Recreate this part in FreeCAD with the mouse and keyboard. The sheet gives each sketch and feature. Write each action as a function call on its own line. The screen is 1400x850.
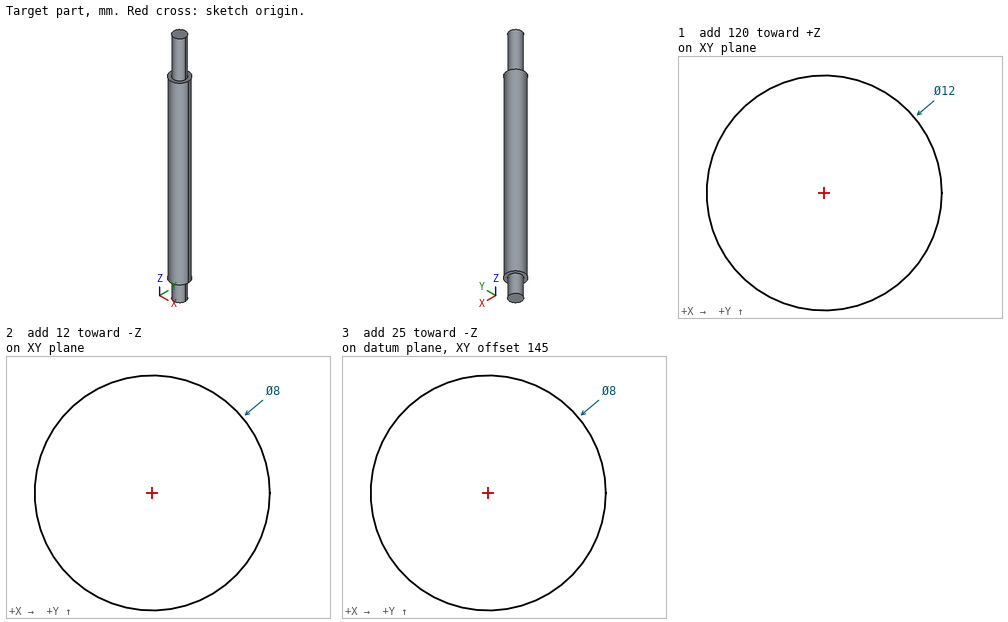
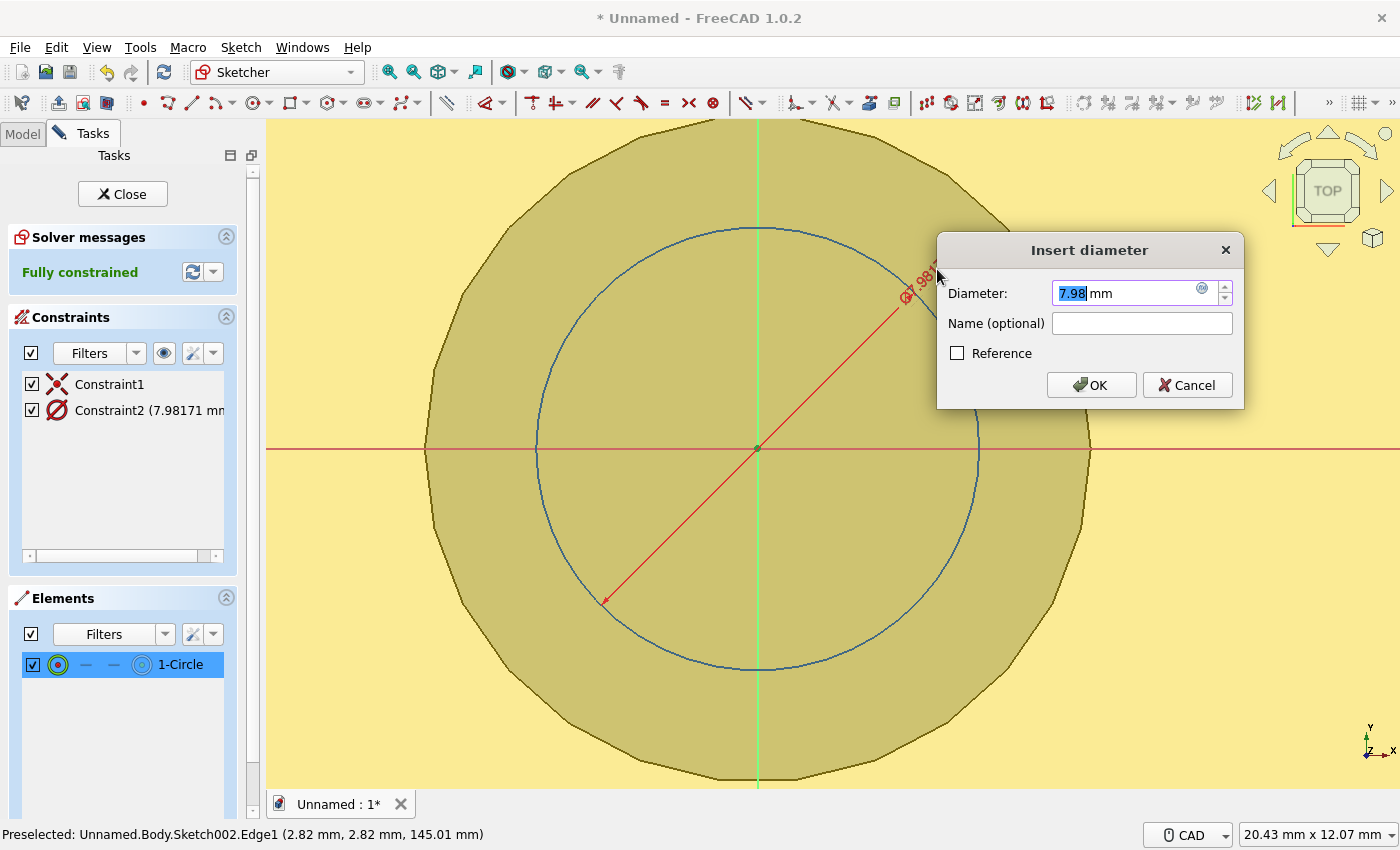
text(8)
key(Return)
key(Escape)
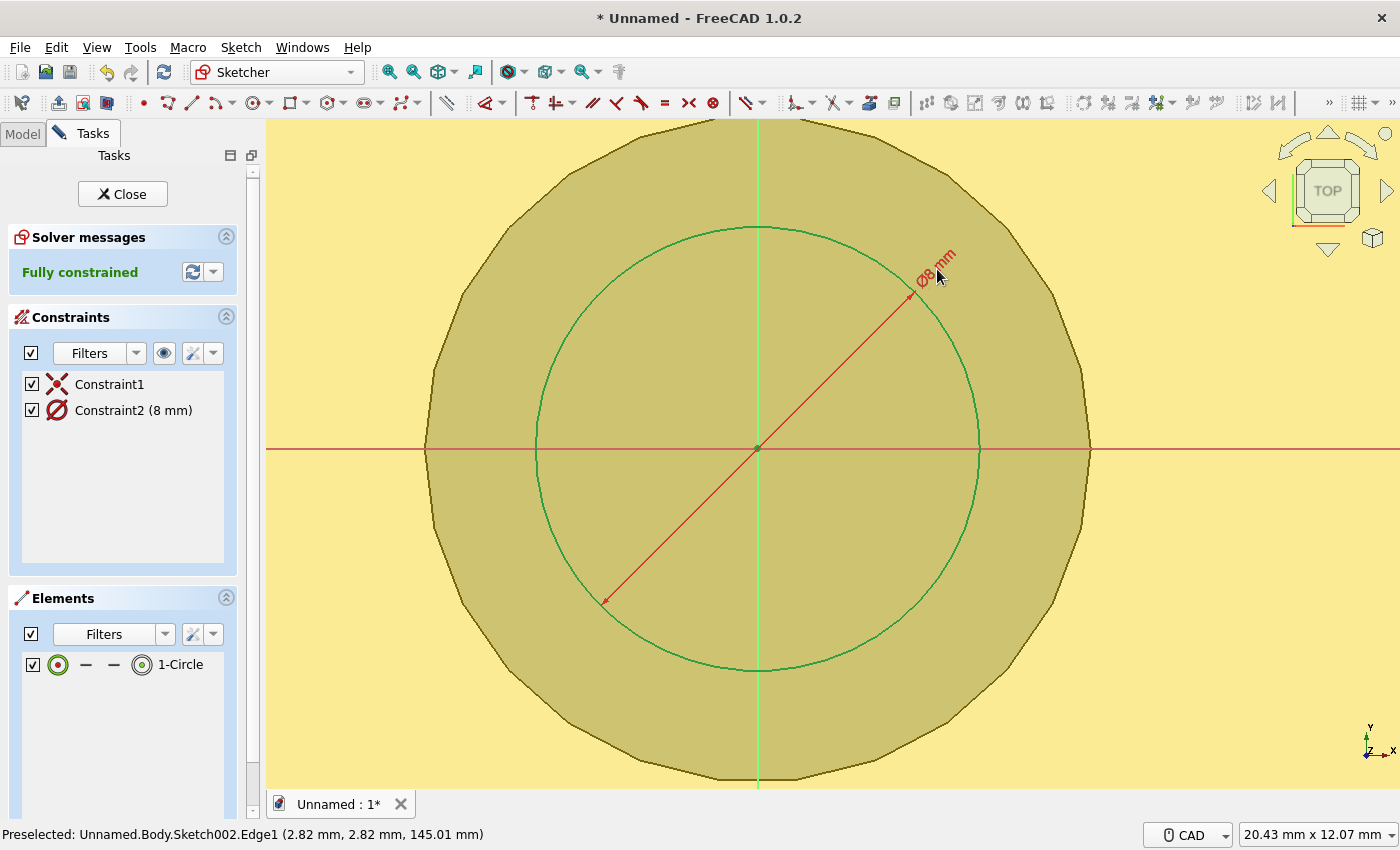
click(123, 194)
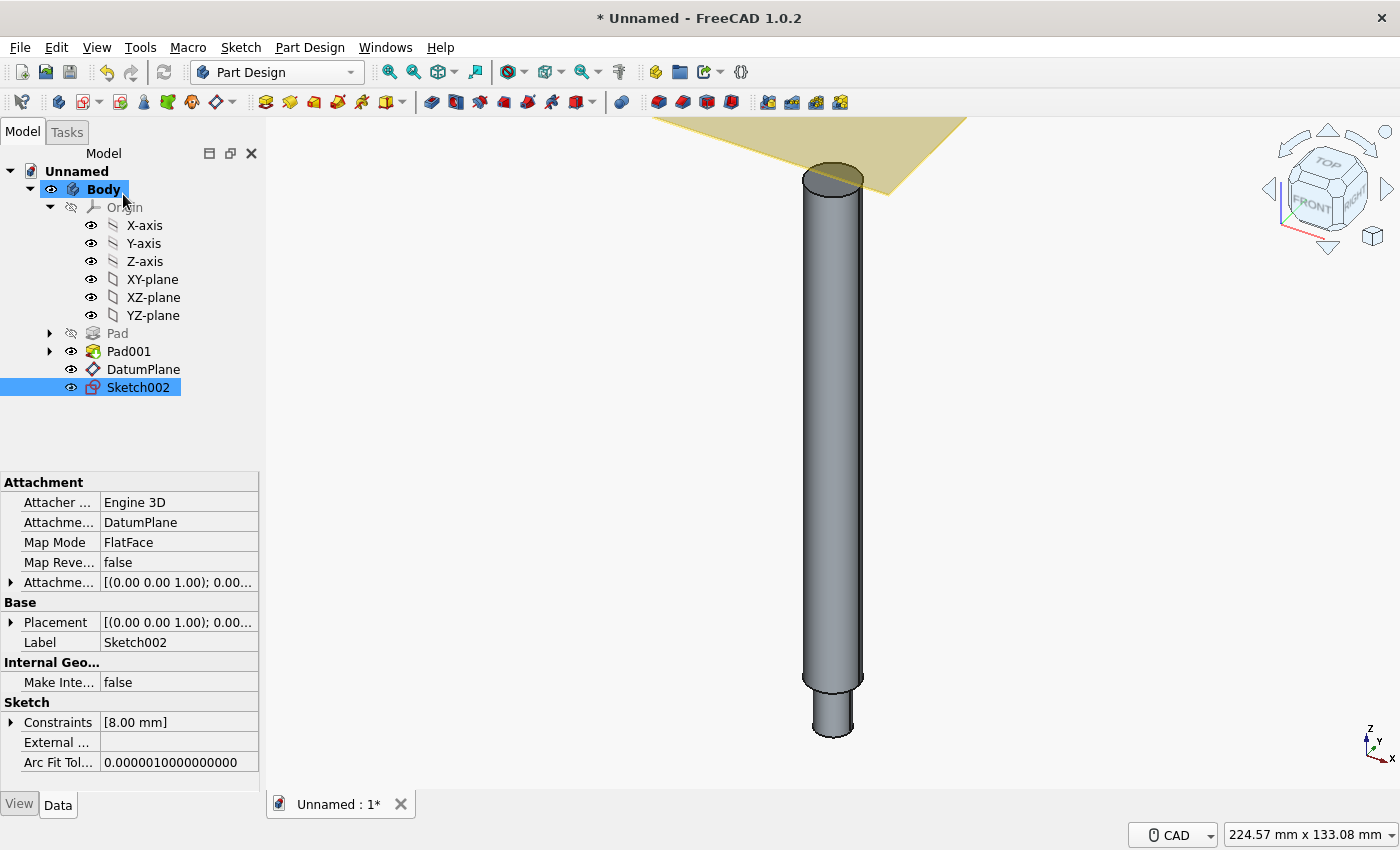
click(266, 102)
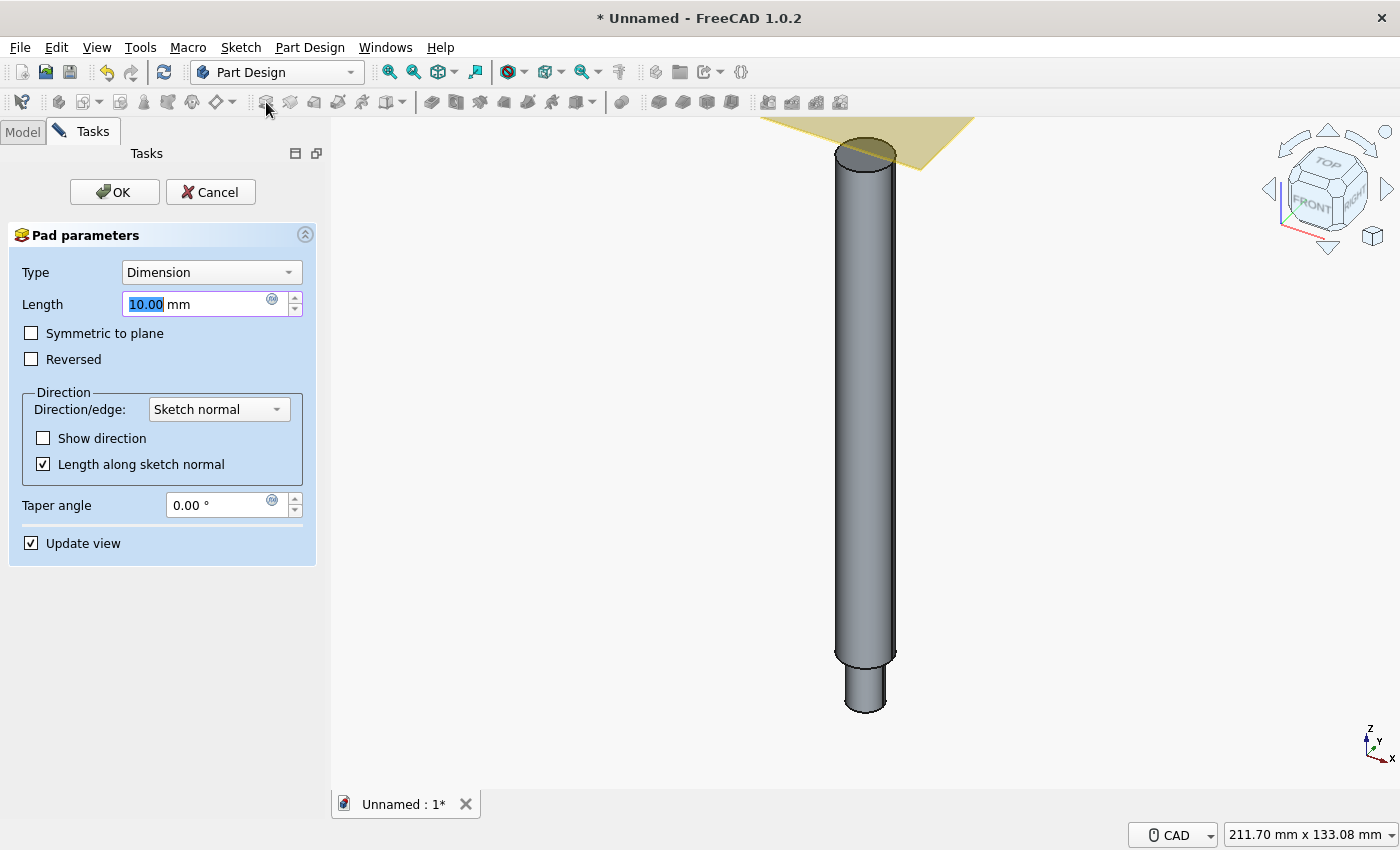
text(25)
key(Tab)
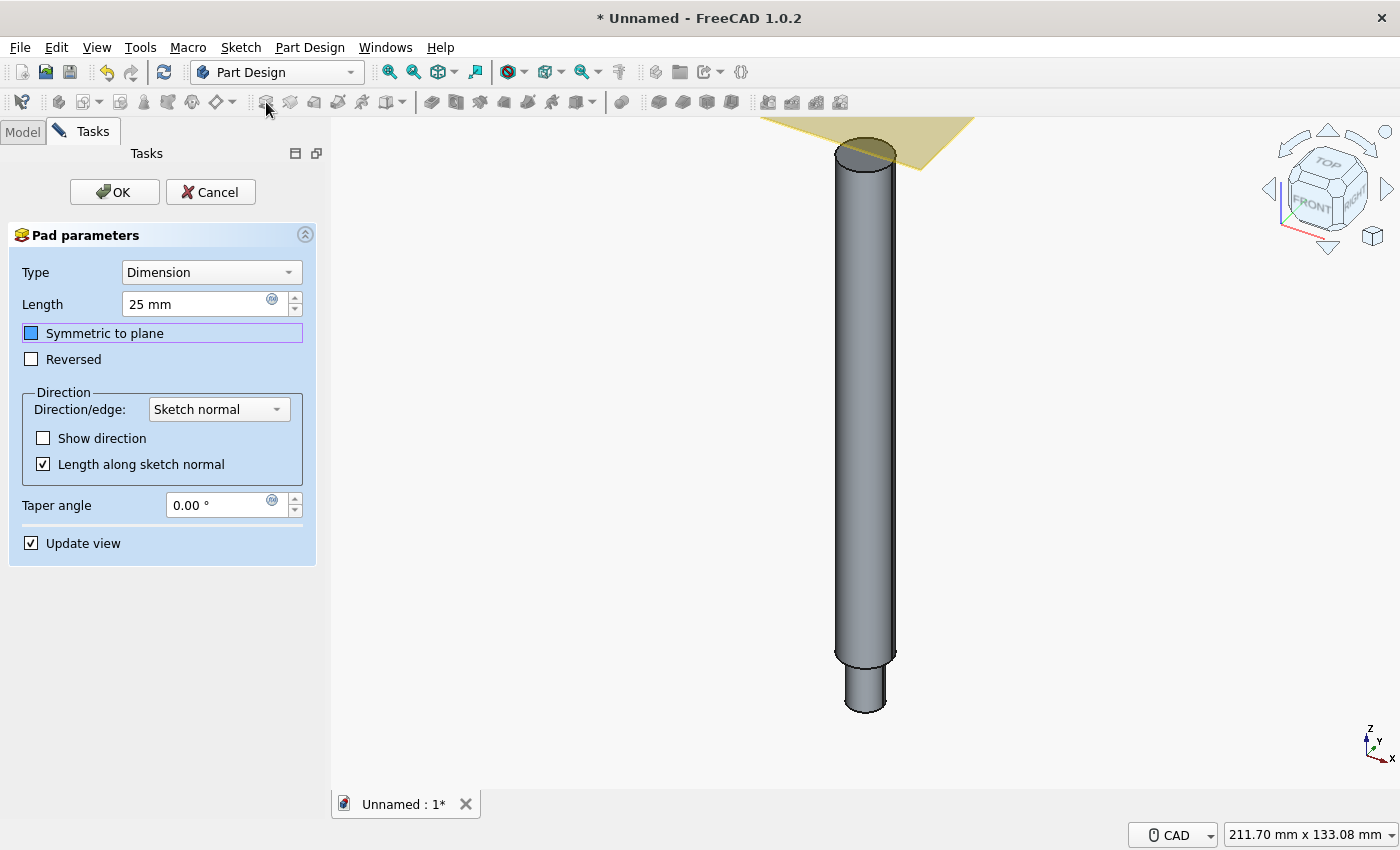
click(30, 359)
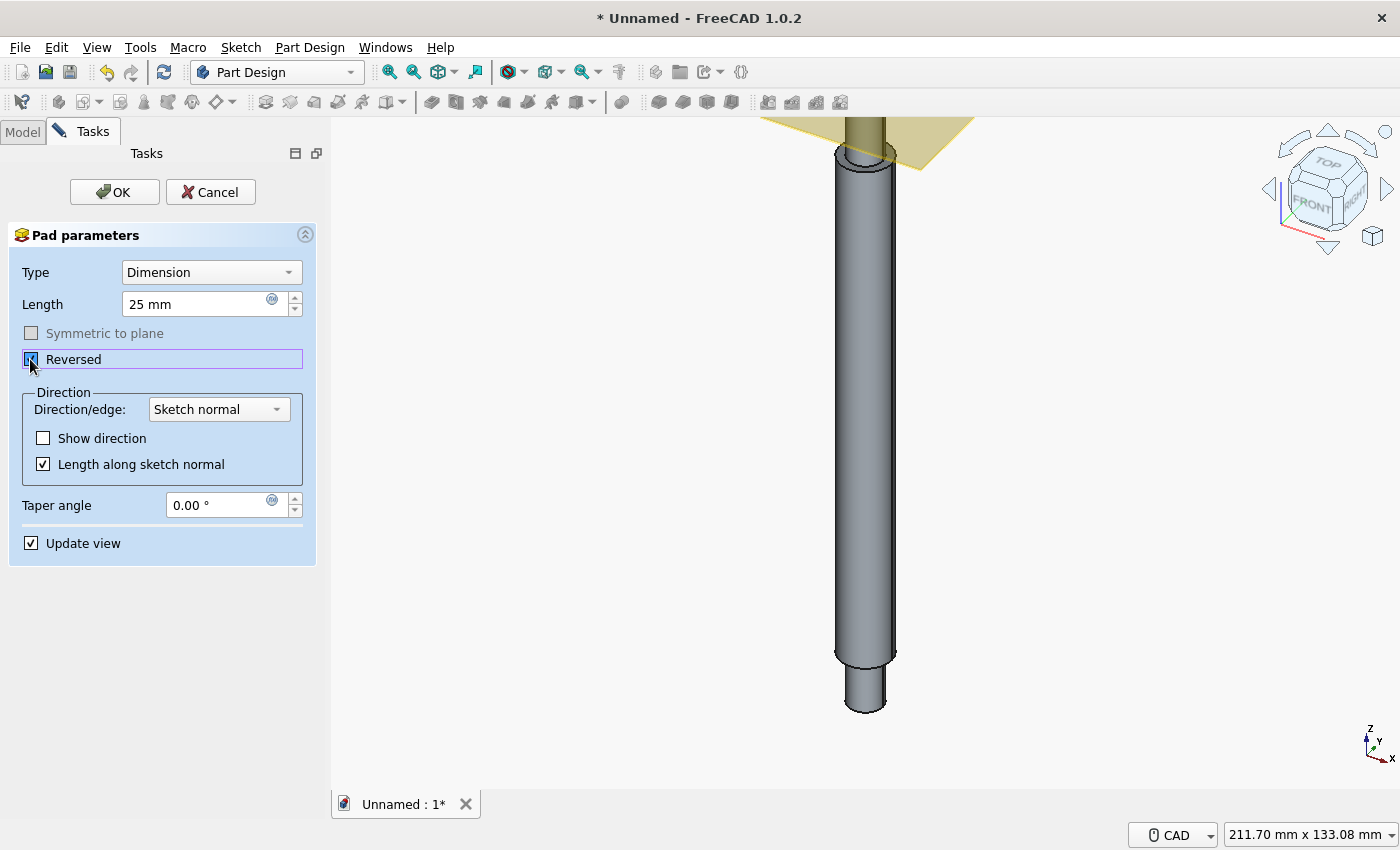
click(115, 192)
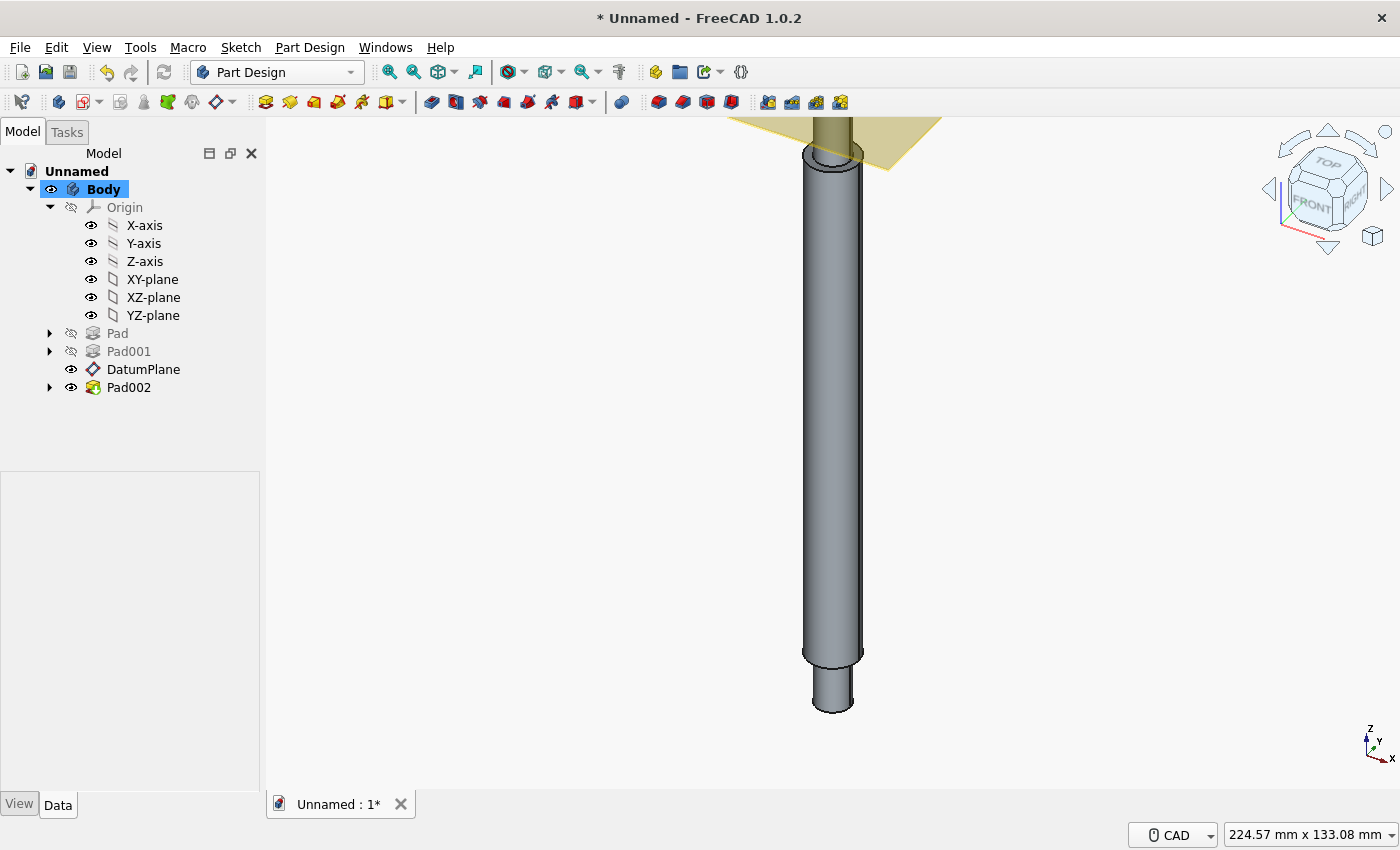
click(116, 369)
key(space)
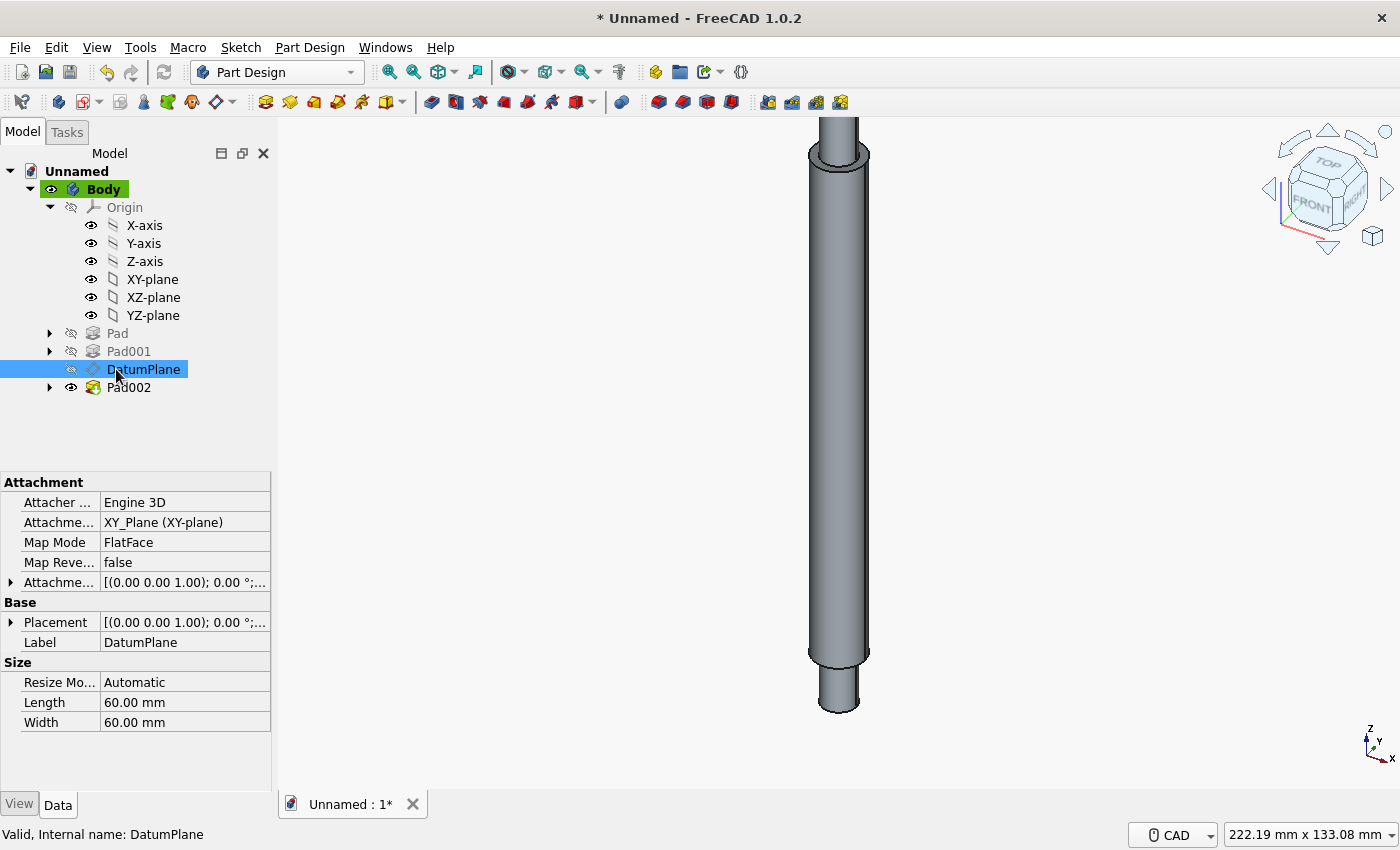
key(0)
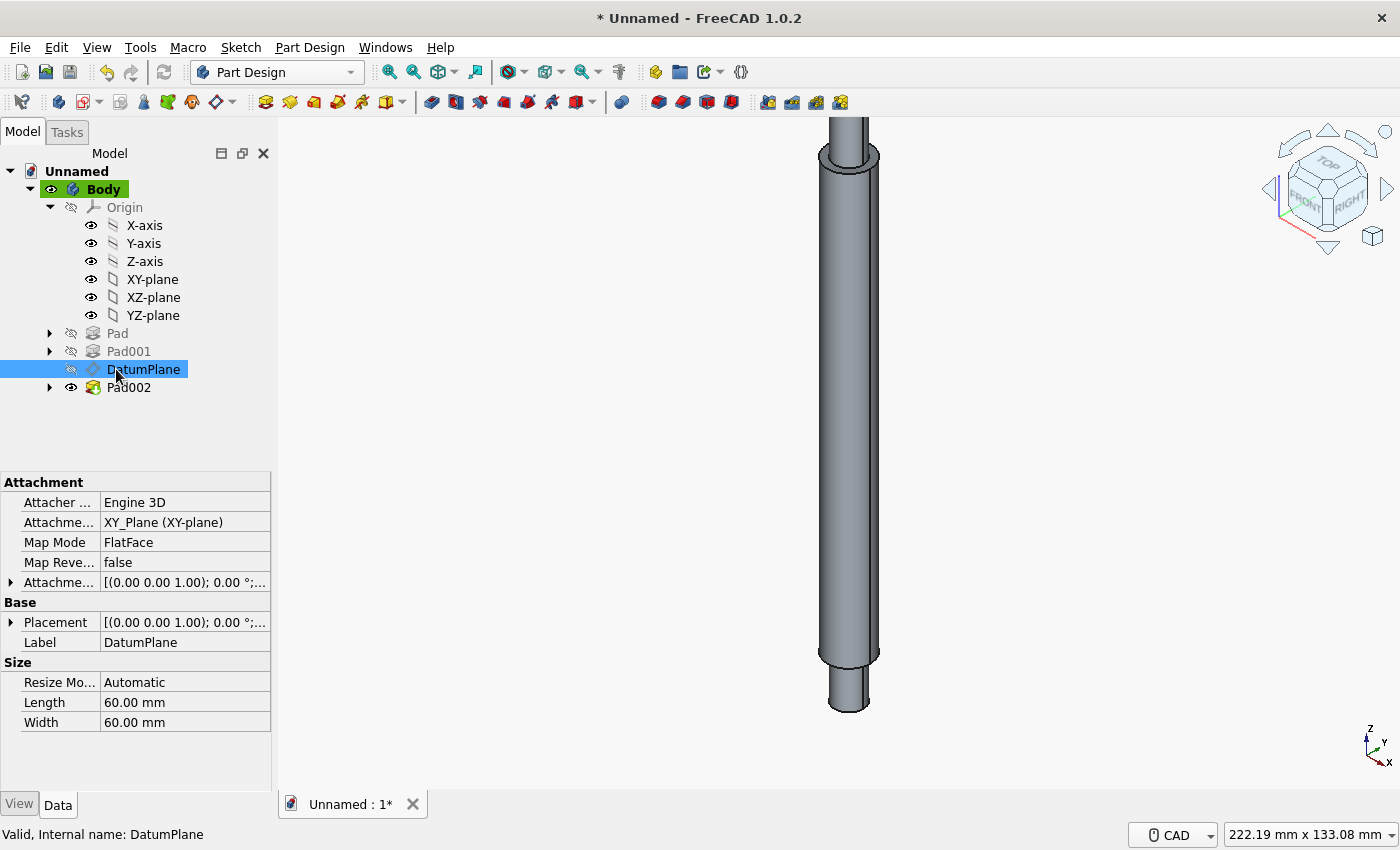
key(v)
key(f)